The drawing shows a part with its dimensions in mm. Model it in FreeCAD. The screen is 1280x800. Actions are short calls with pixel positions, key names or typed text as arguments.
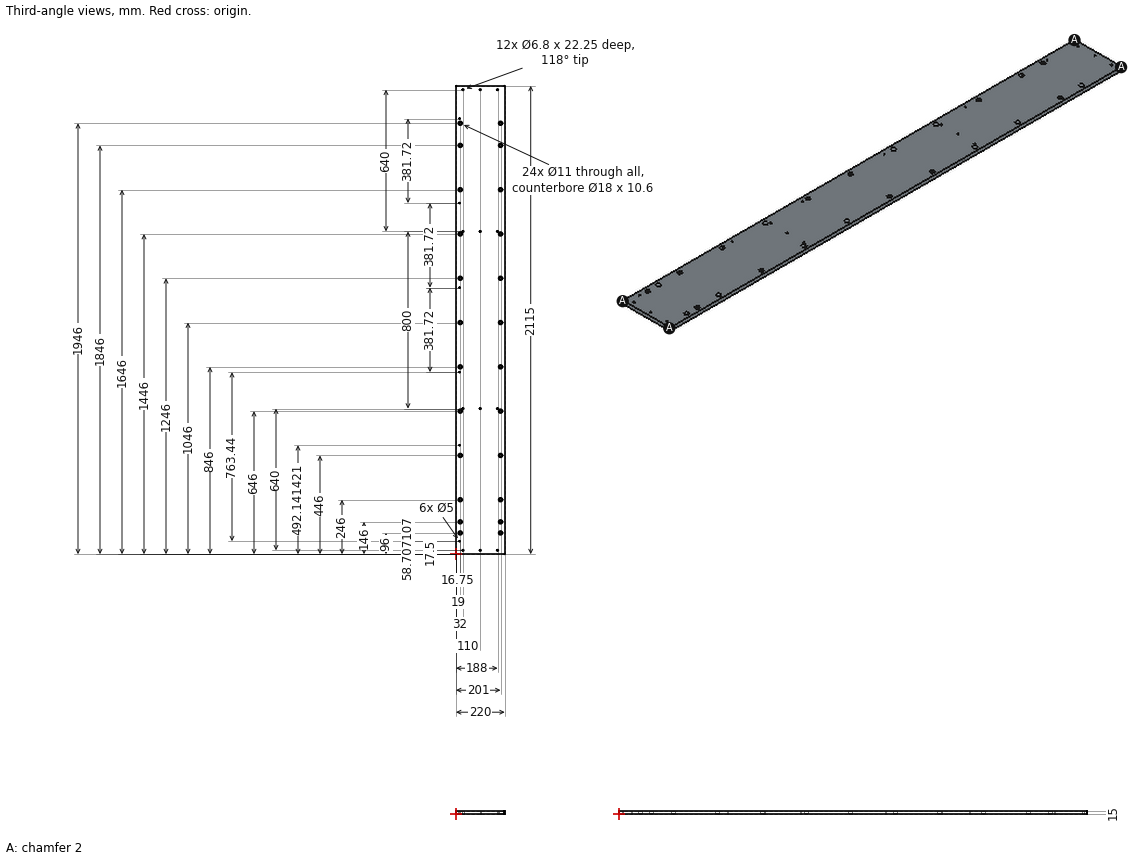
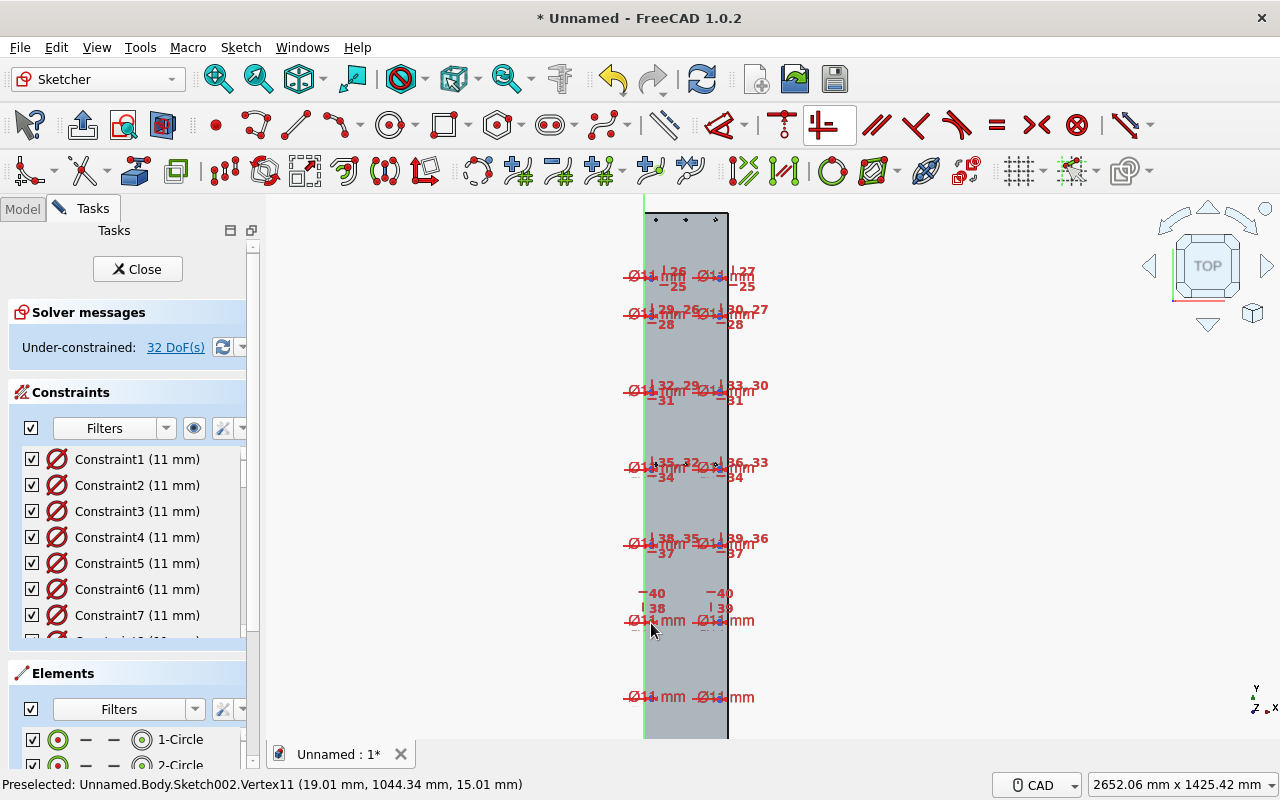
click(651, 699)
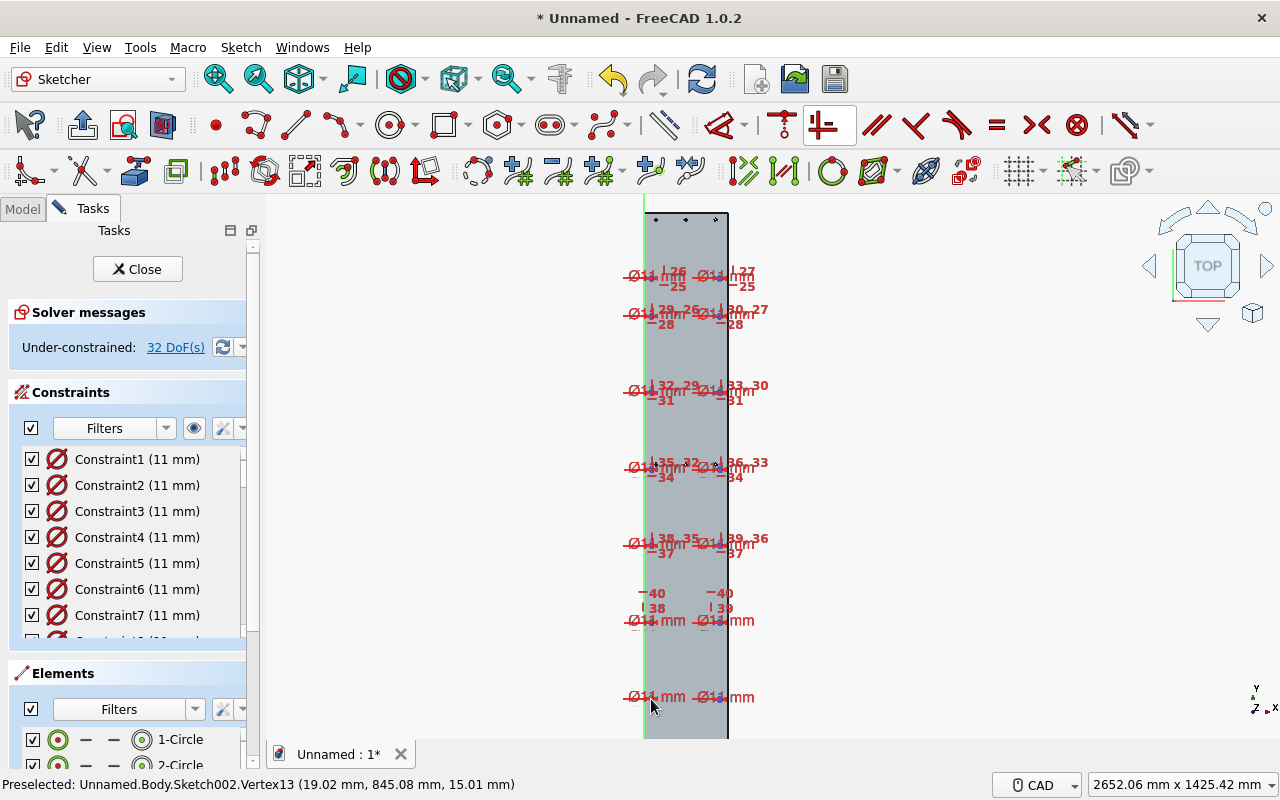
click(850, 126)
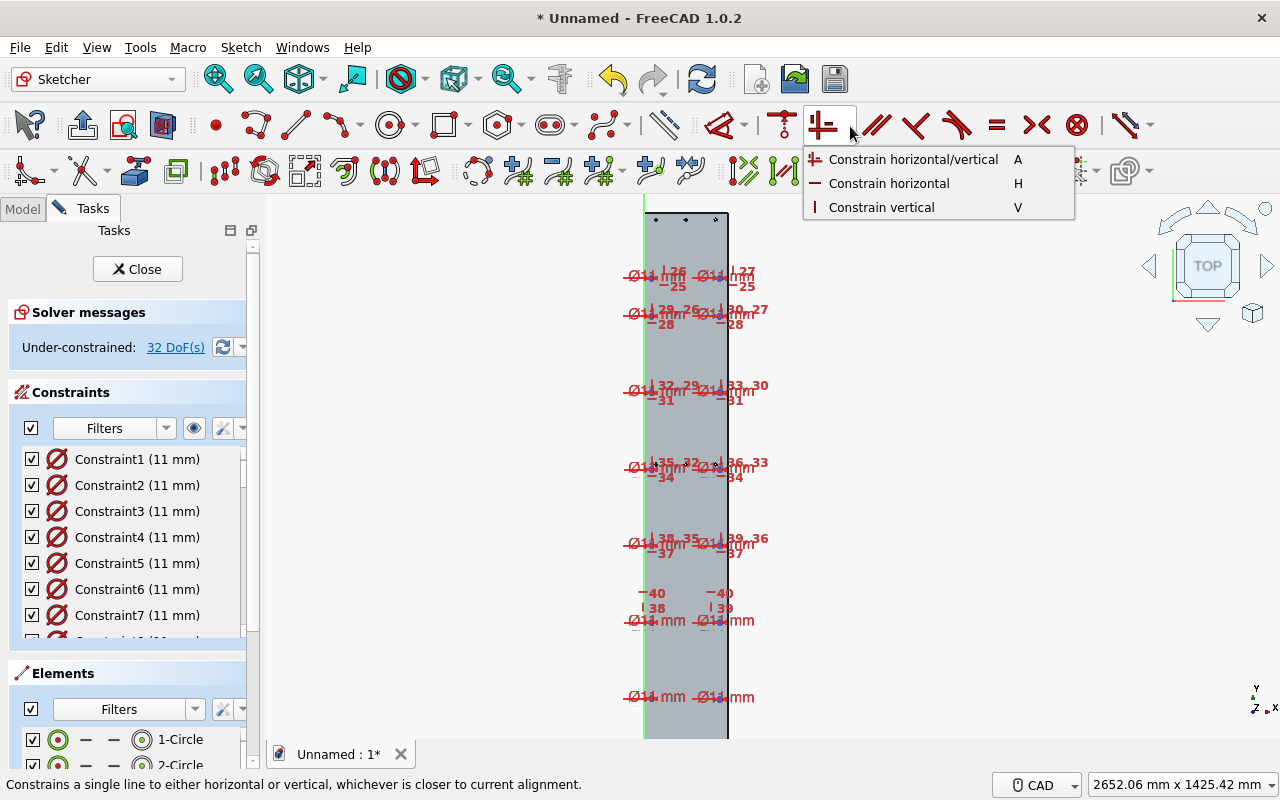
click(939, 207)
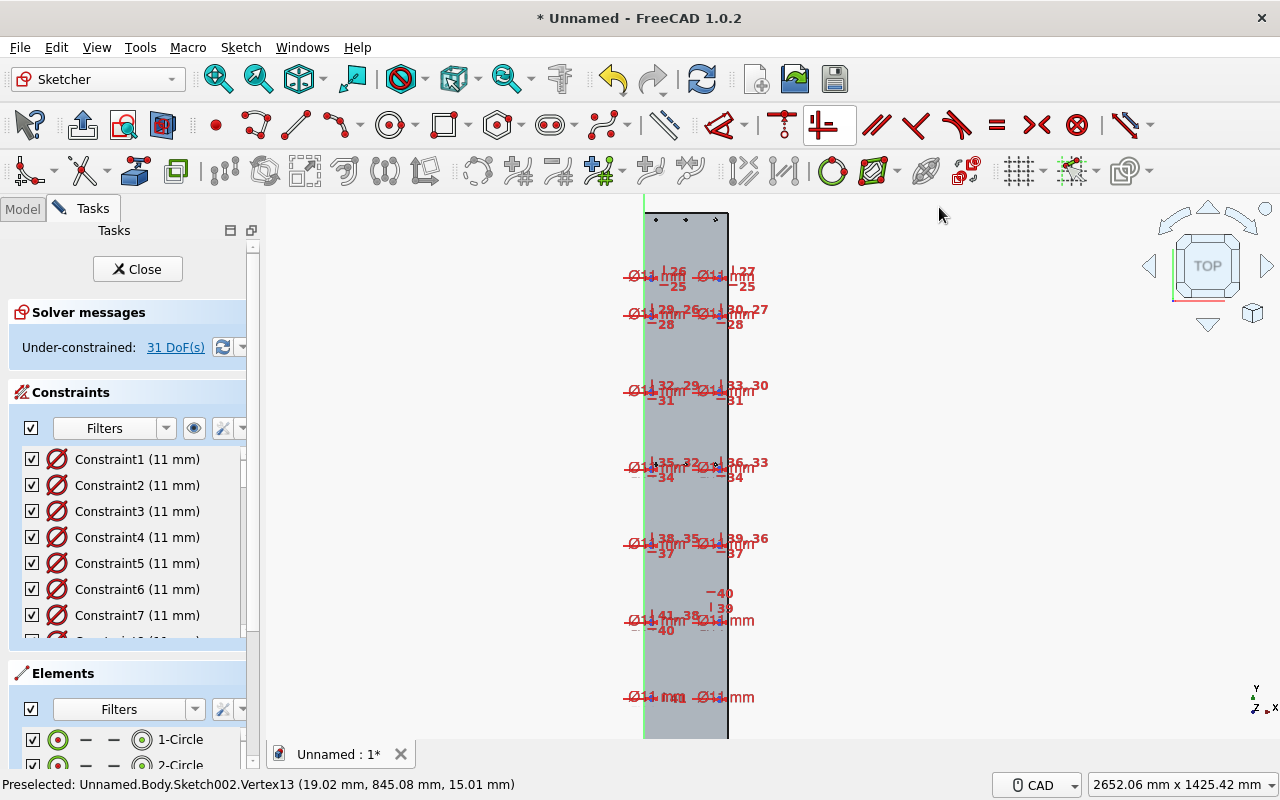
click(720, 623)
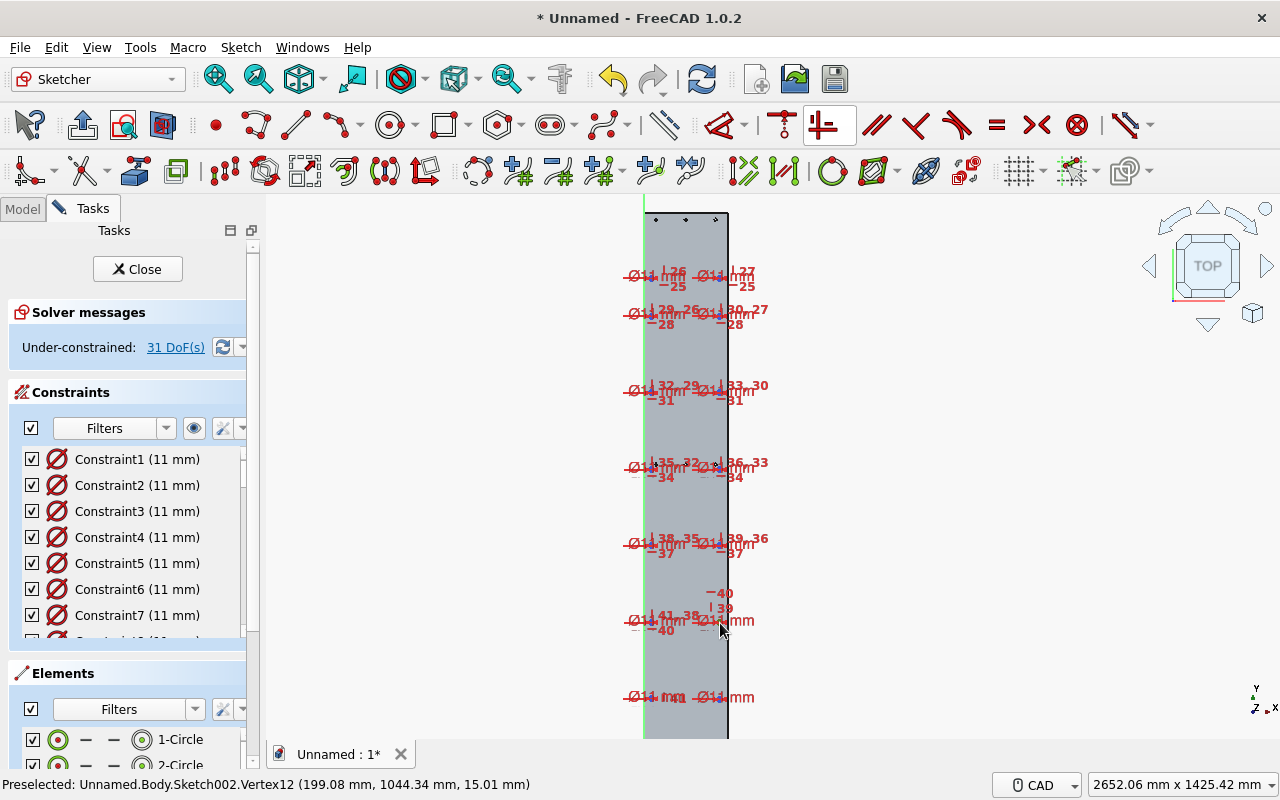
click(720, 699)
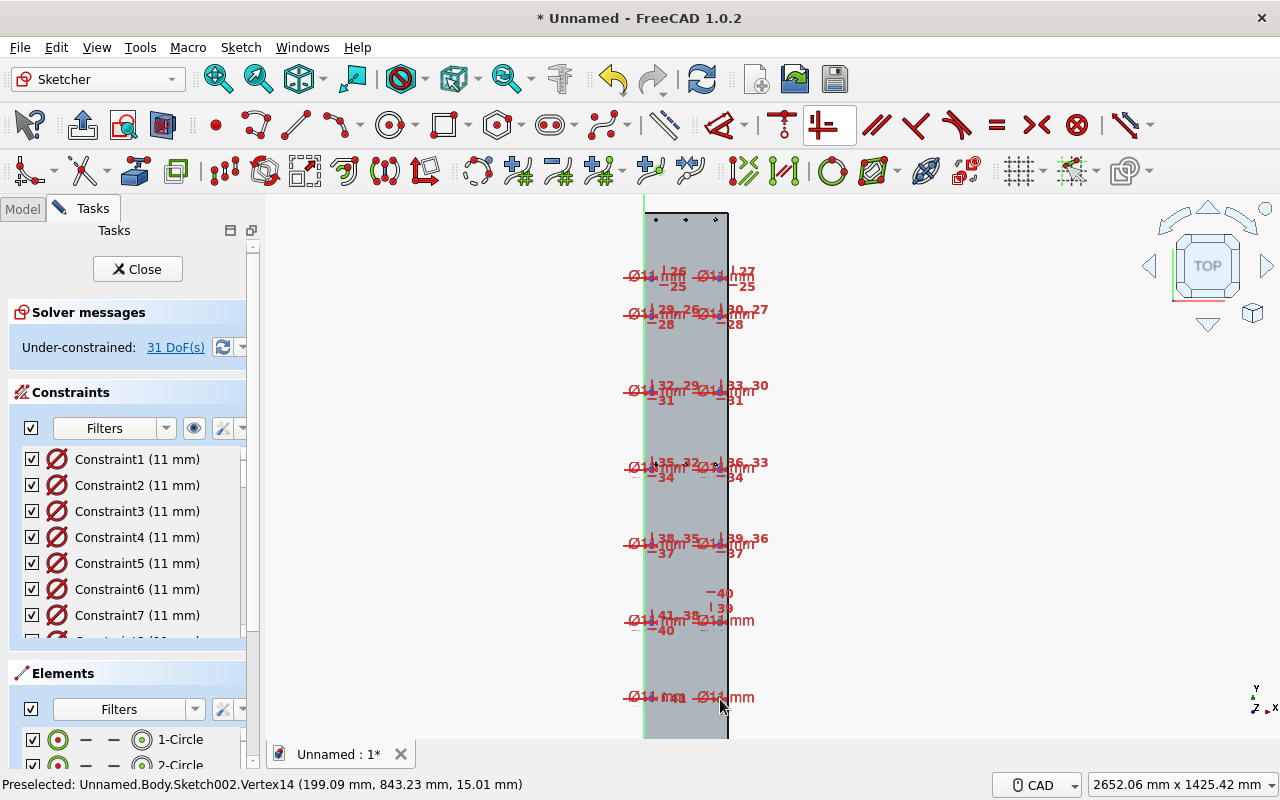
key(v)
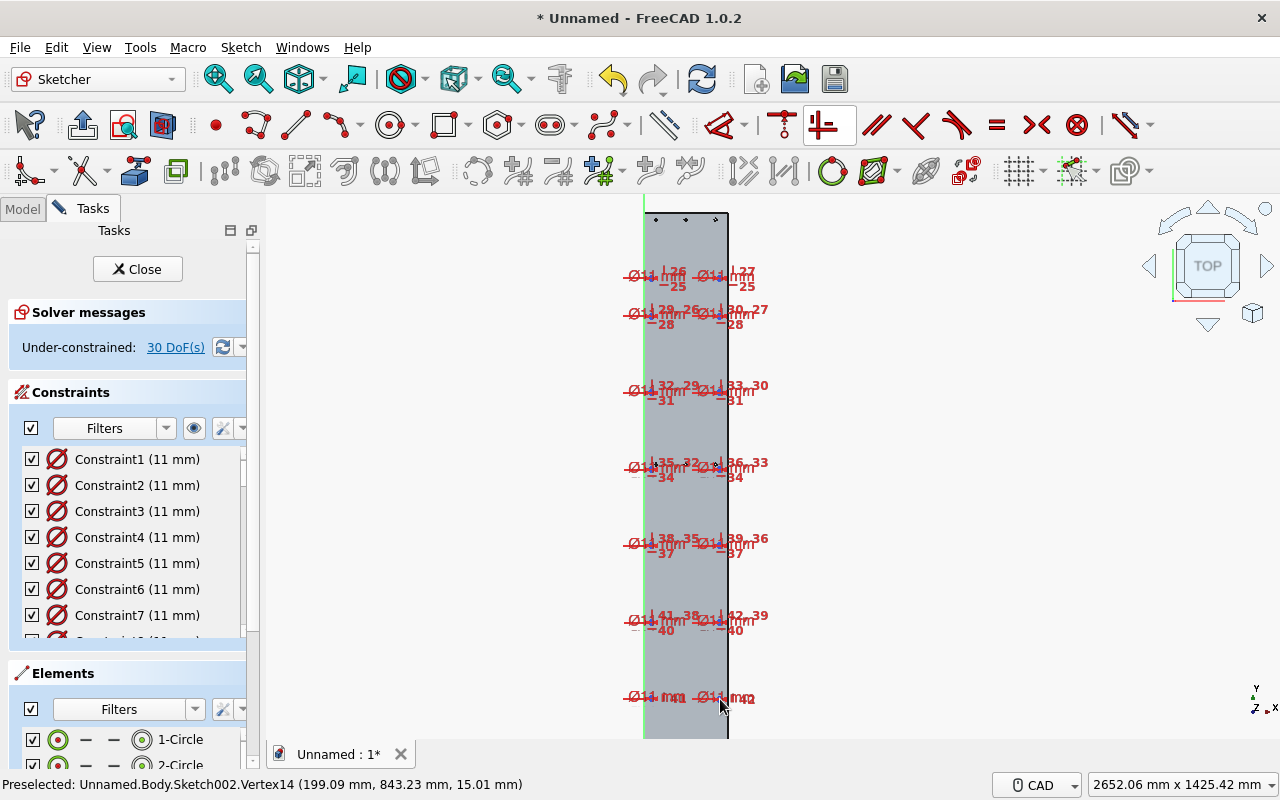
click(651, 699)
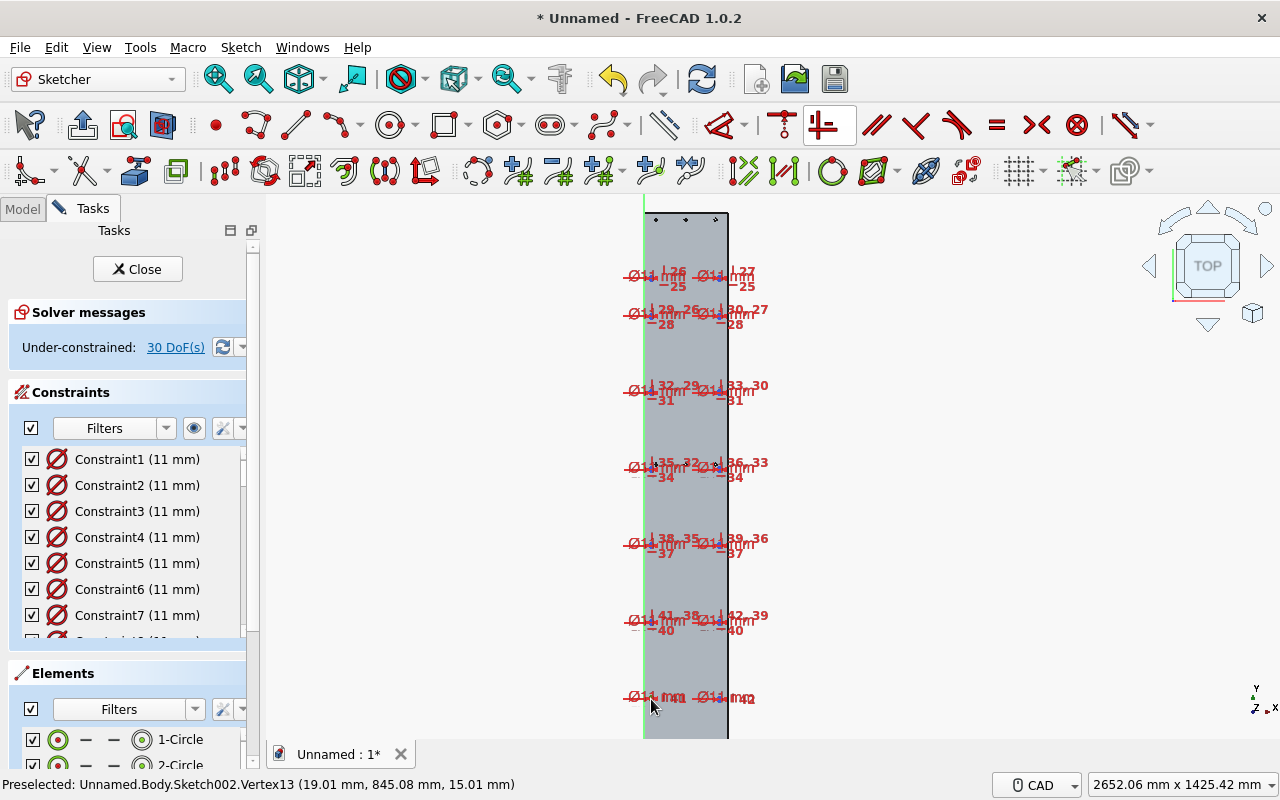
click(720, 699)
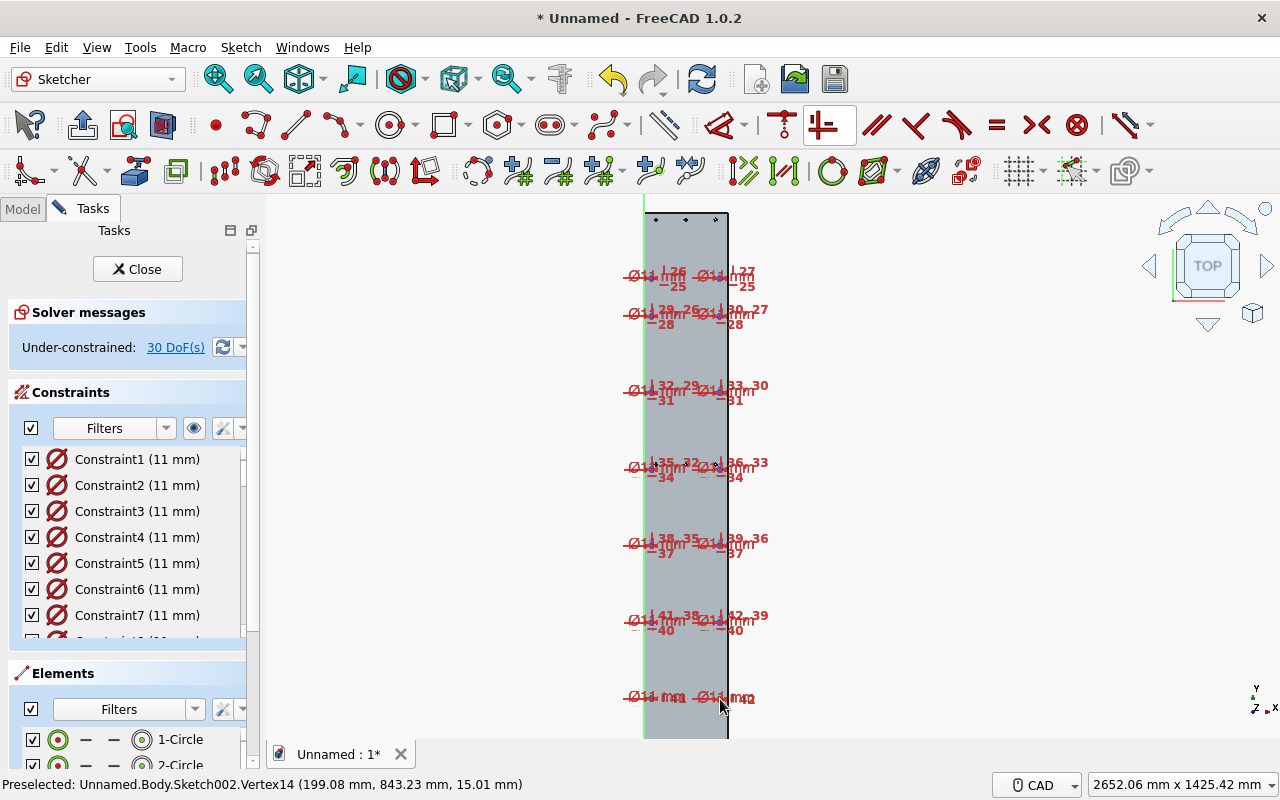
key(h)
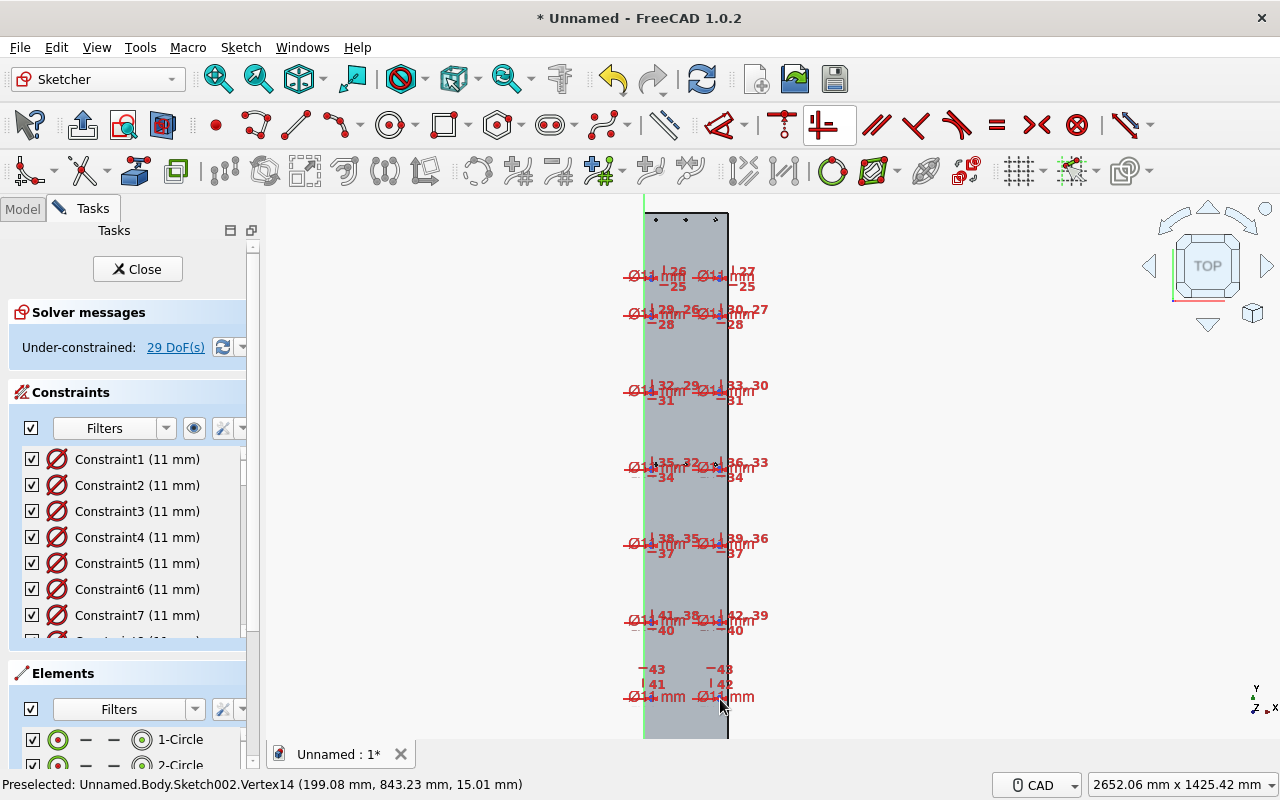
click(651, 699)